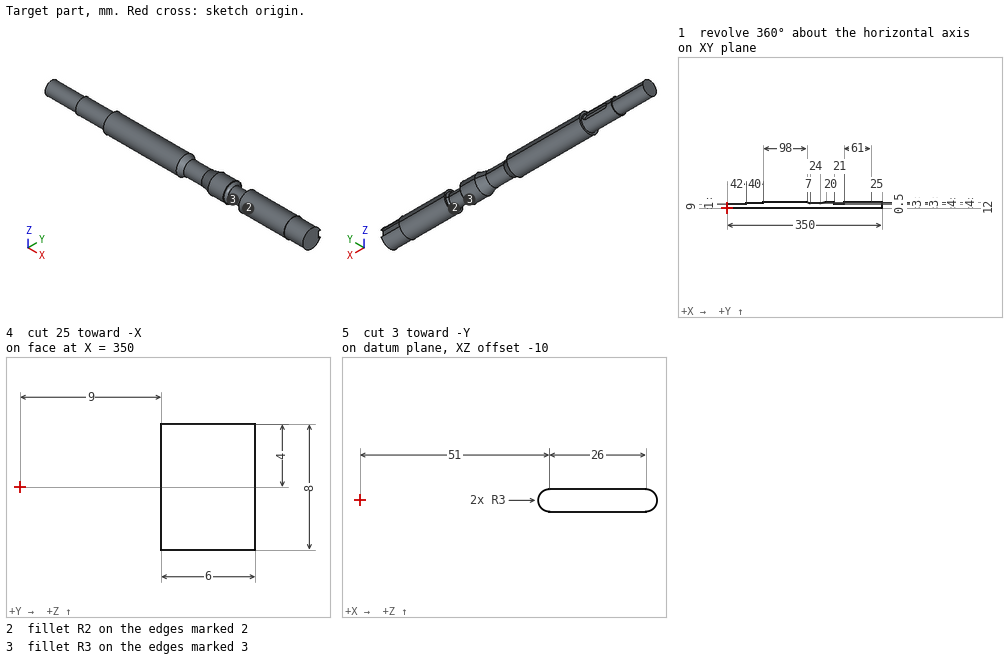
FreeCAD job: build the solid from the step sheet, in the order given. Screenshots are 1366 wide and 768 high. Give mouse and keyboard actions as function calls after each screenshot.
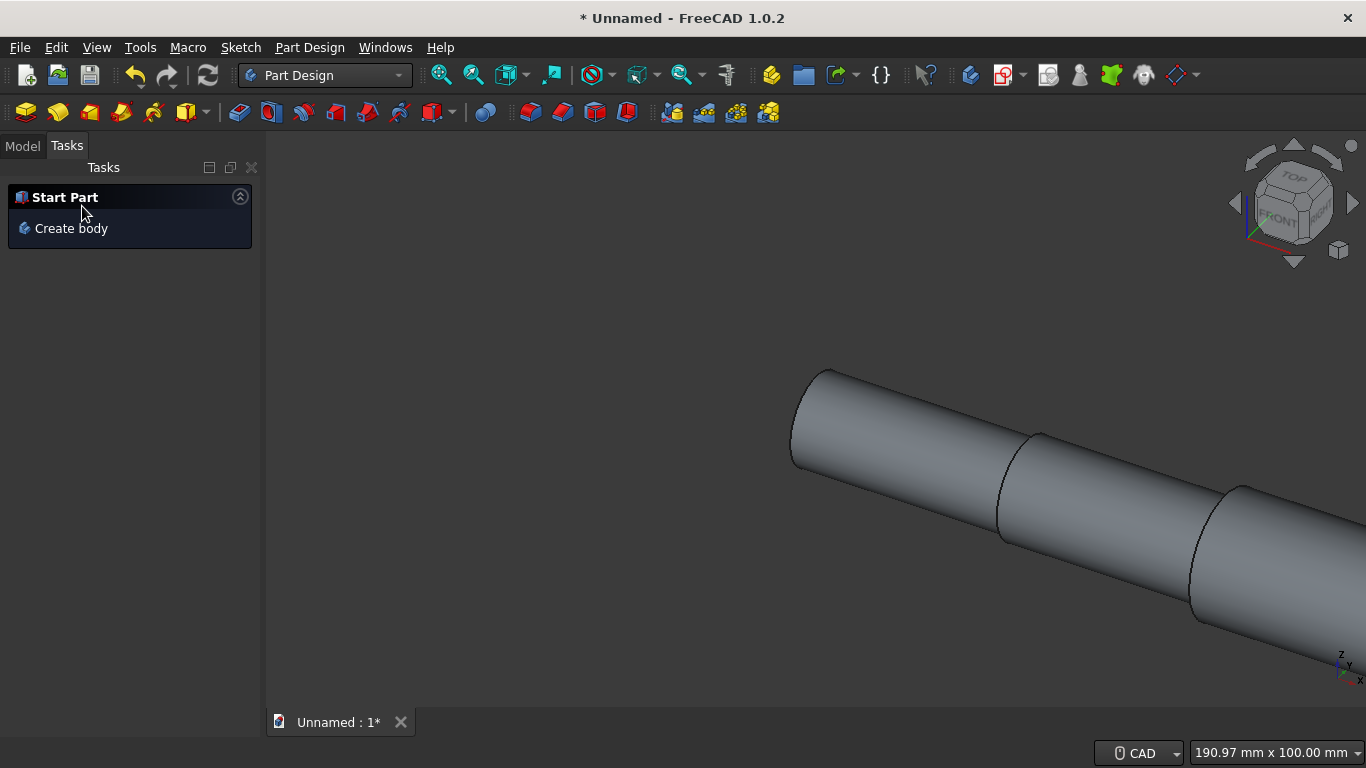
click(442, 76)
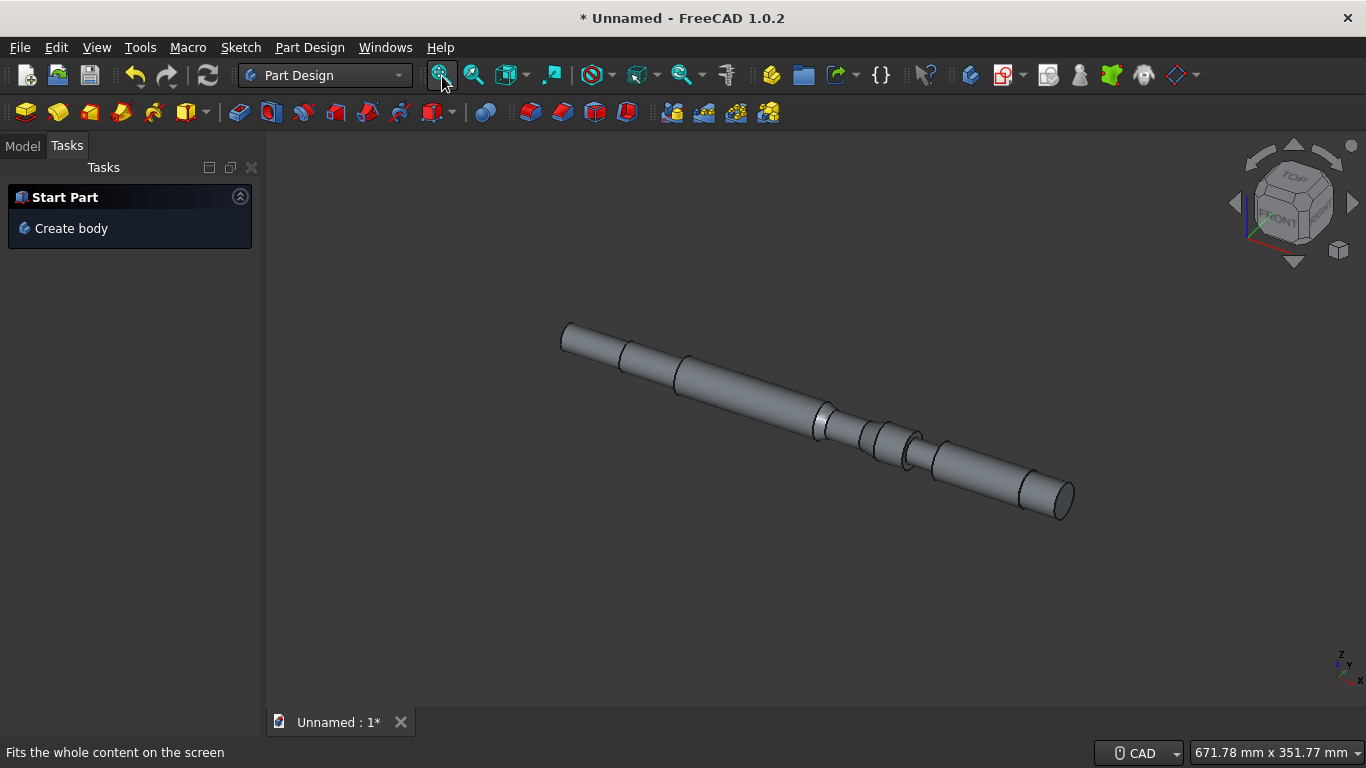
key(0)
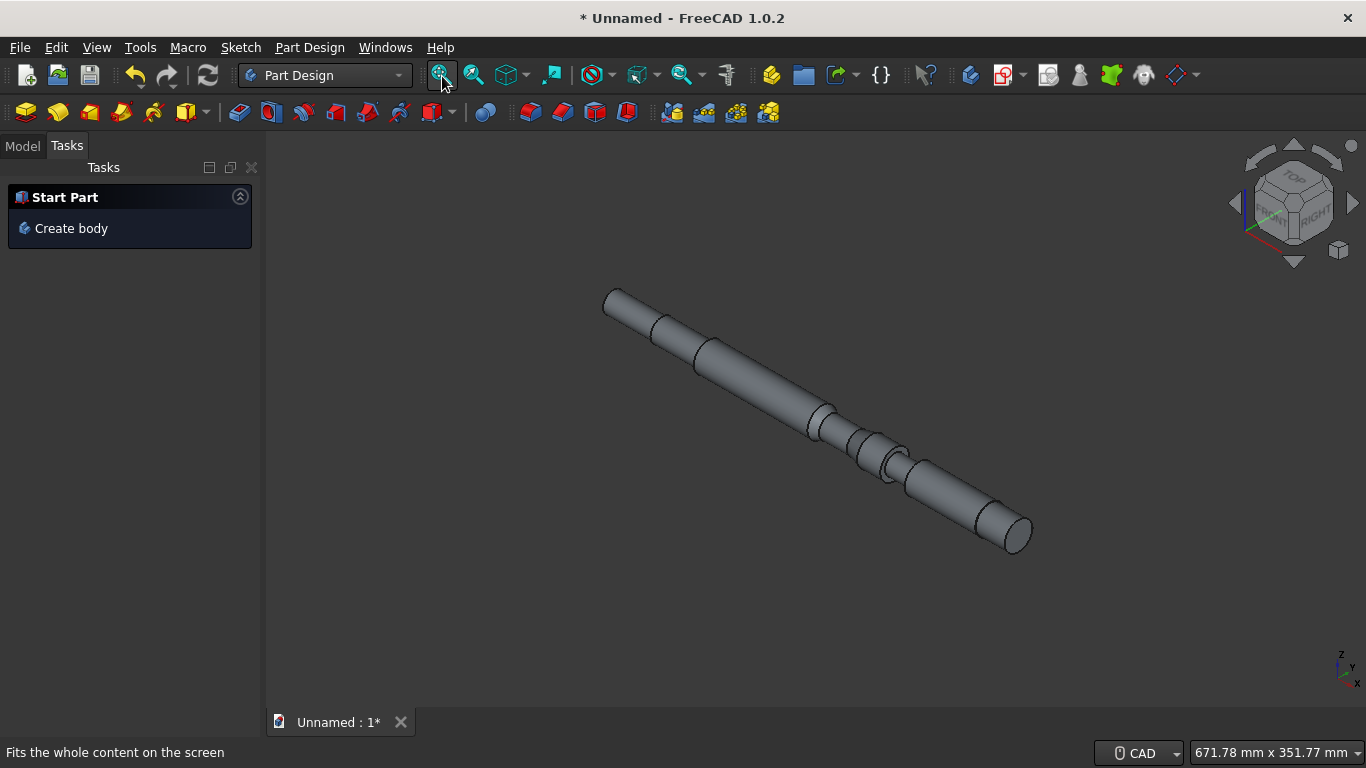
key(2)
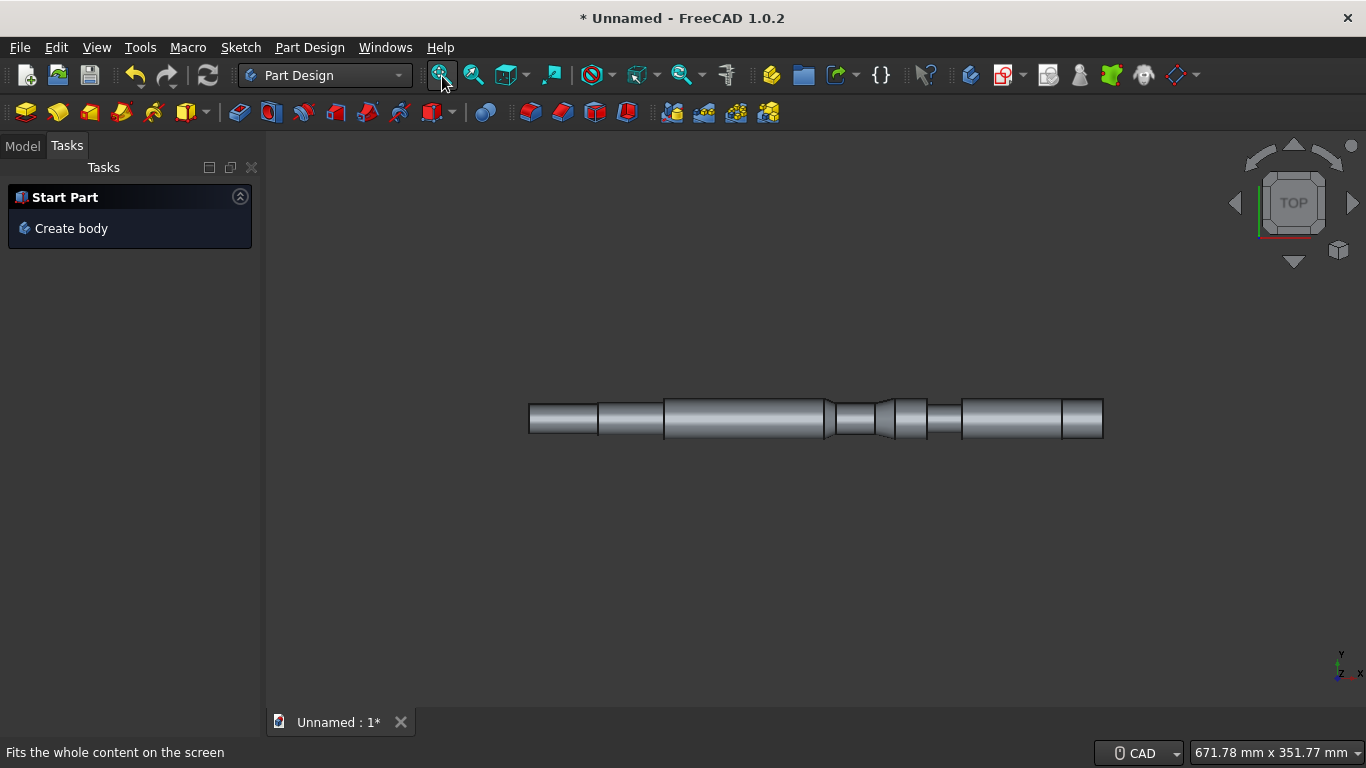
key(1)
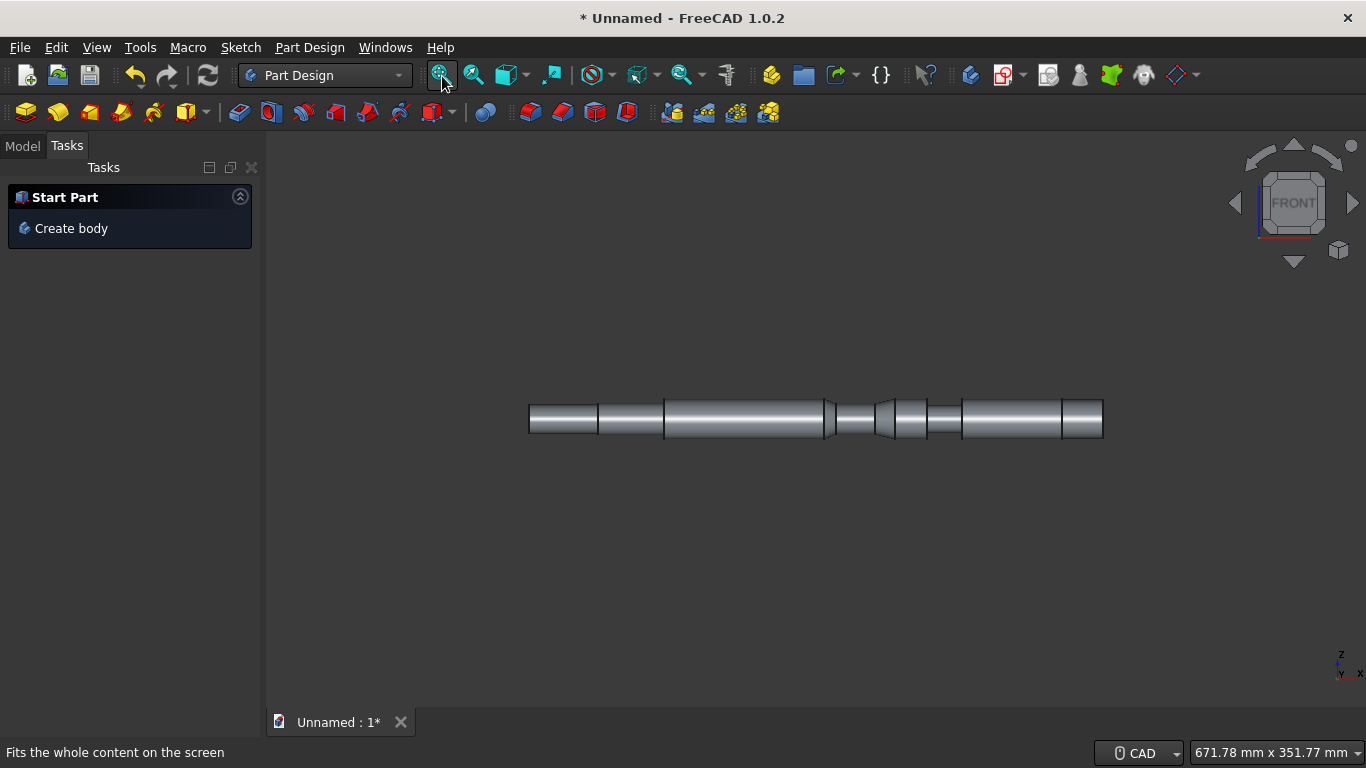
key(3)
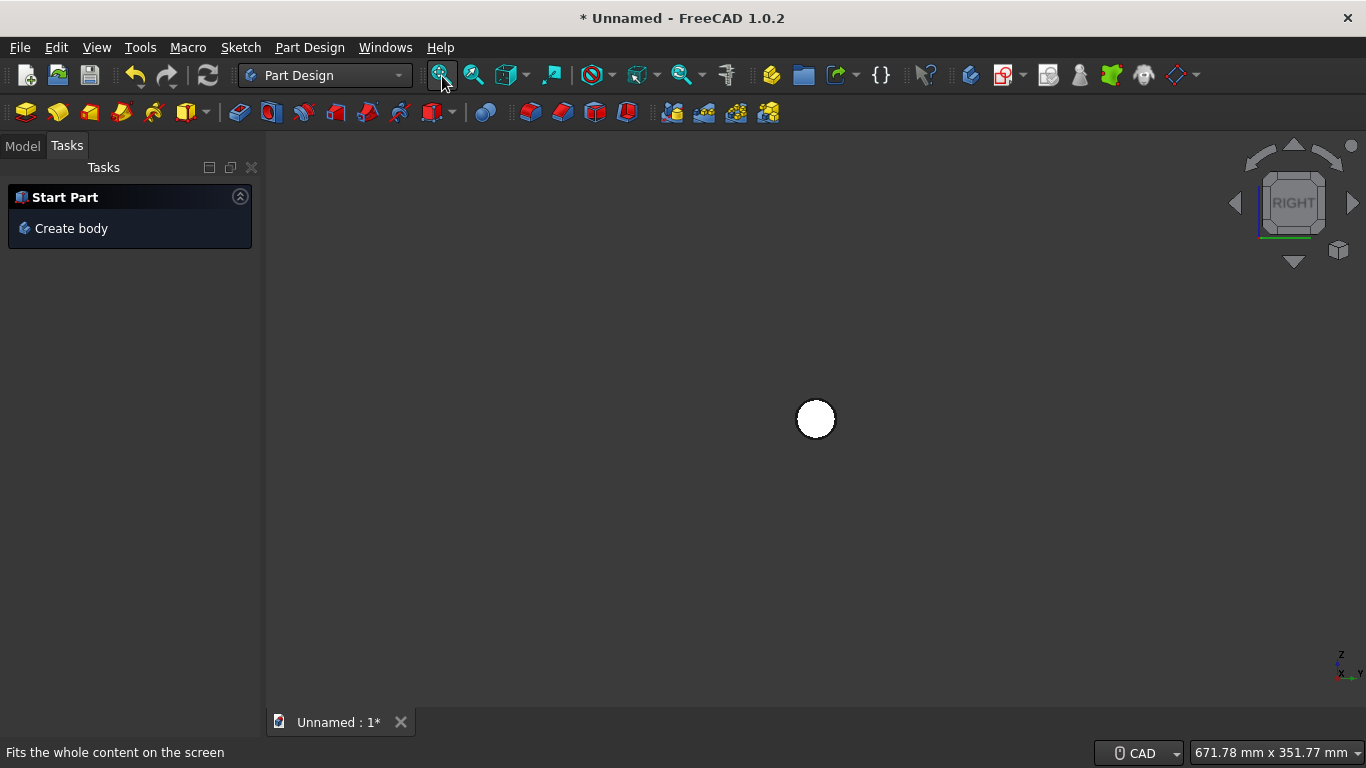
click(442, 76)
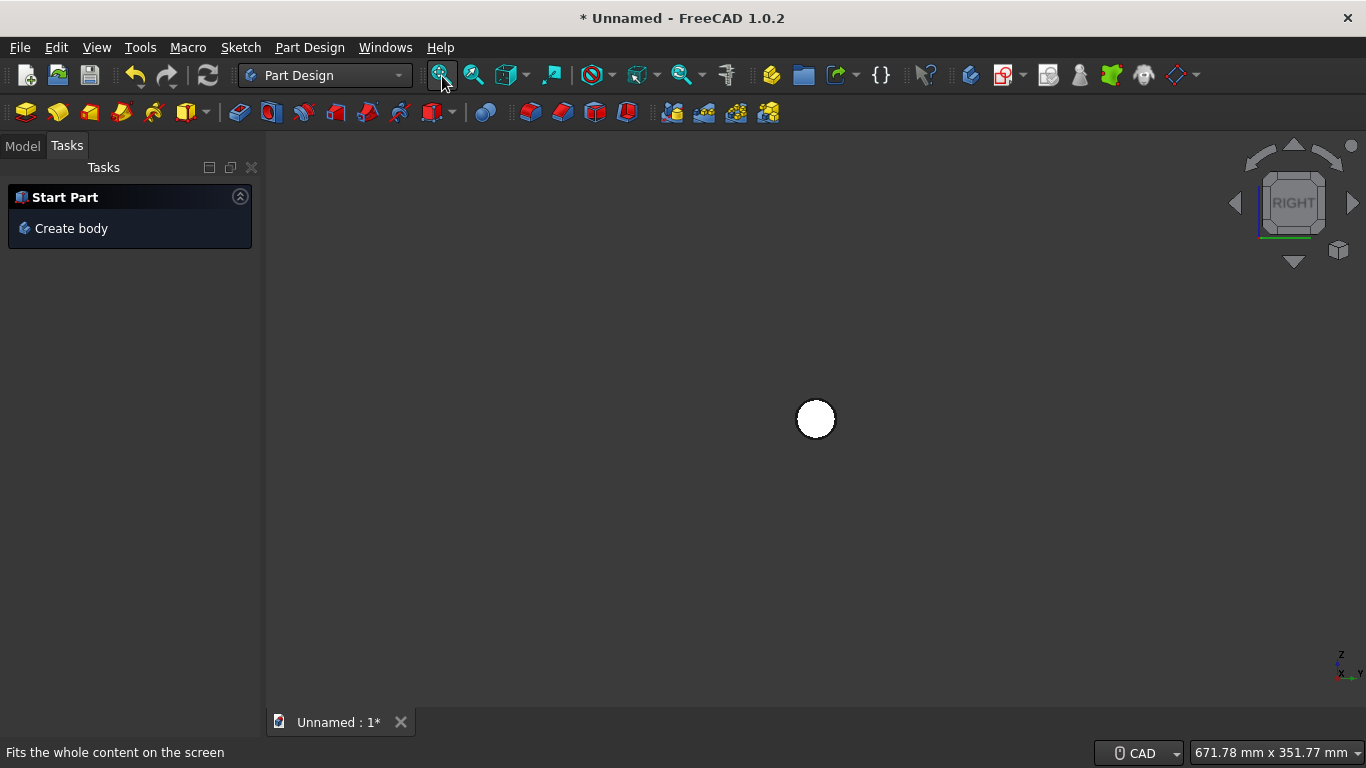
key(5)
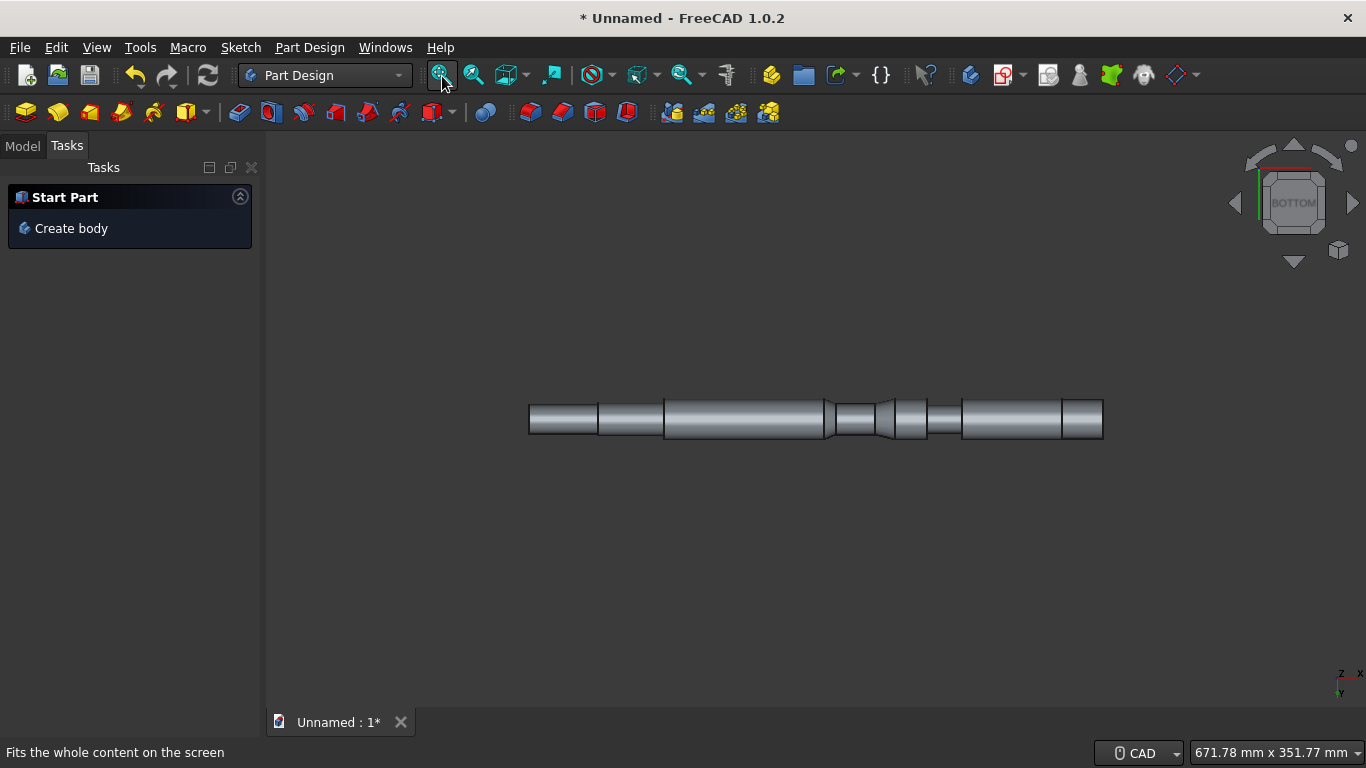
key(4)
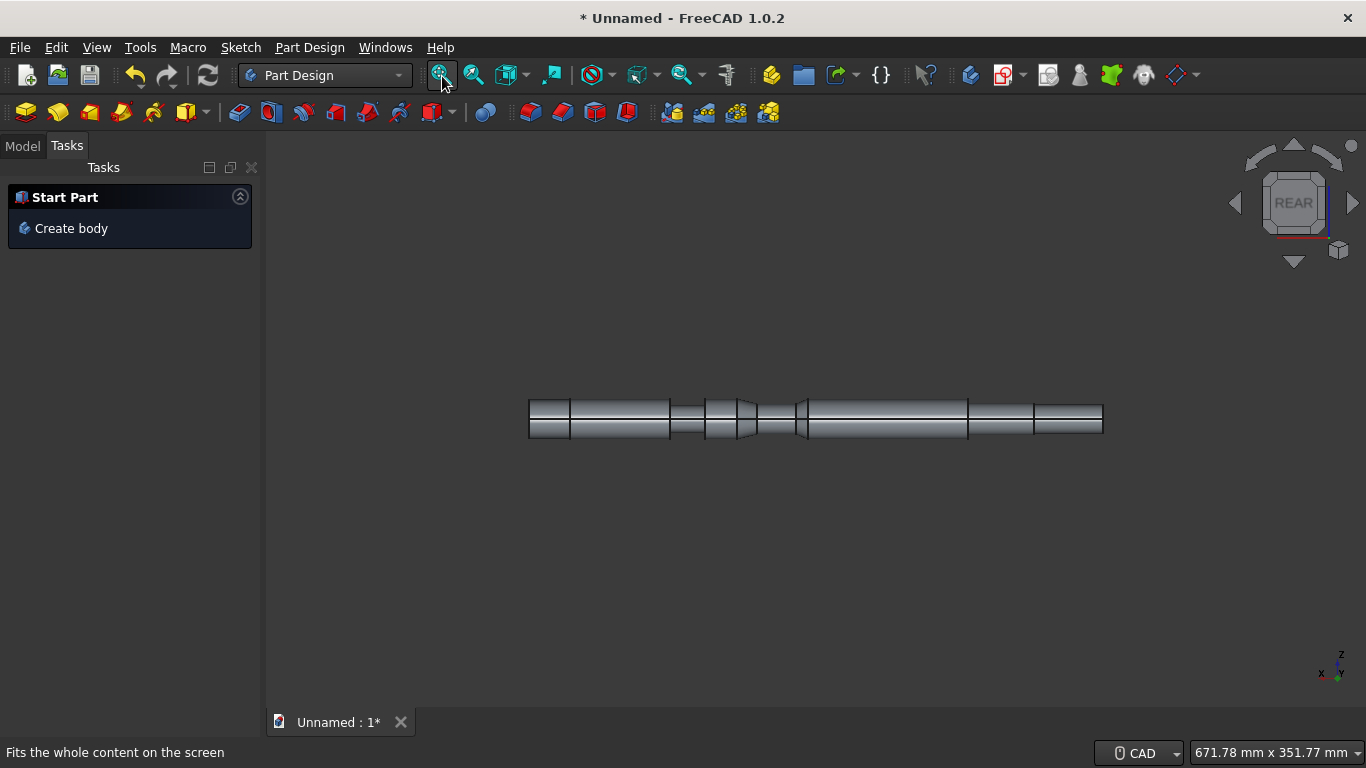
key(6)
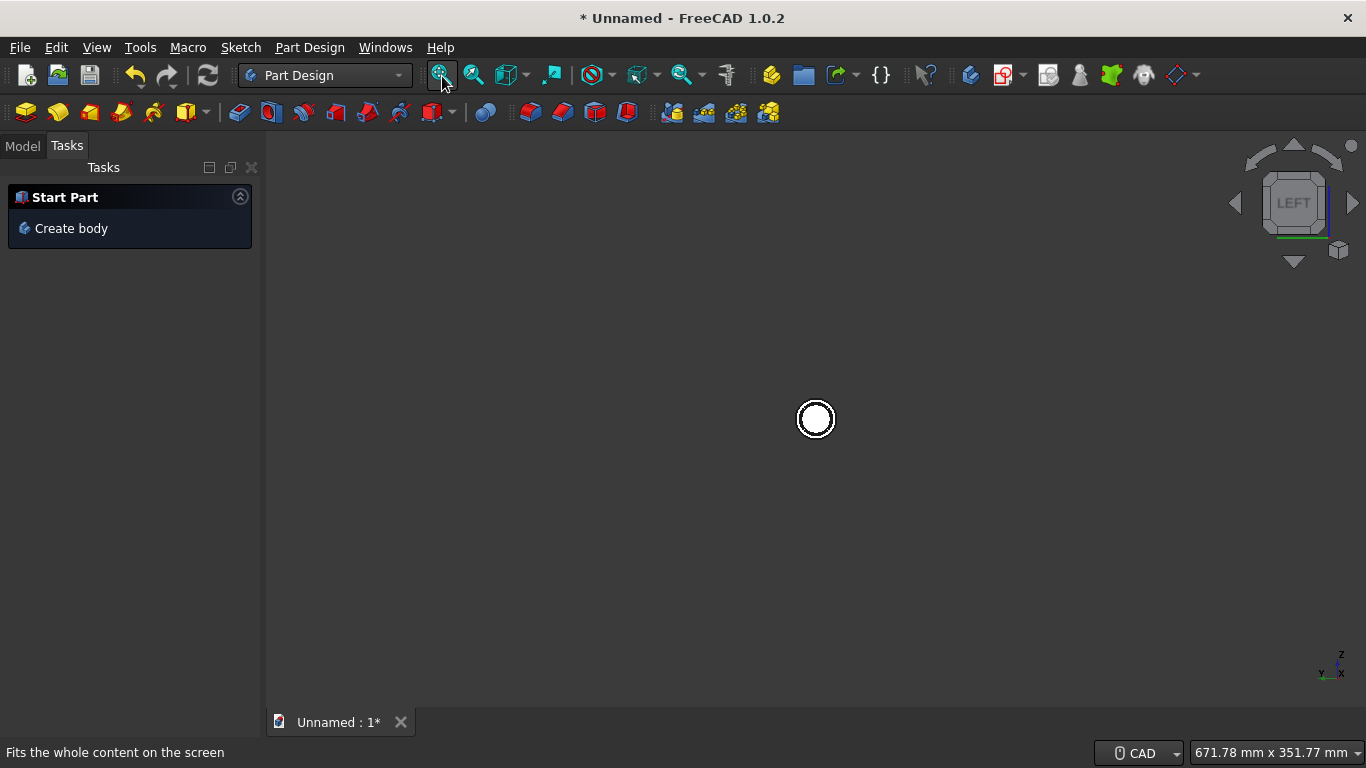
click(442, 76)